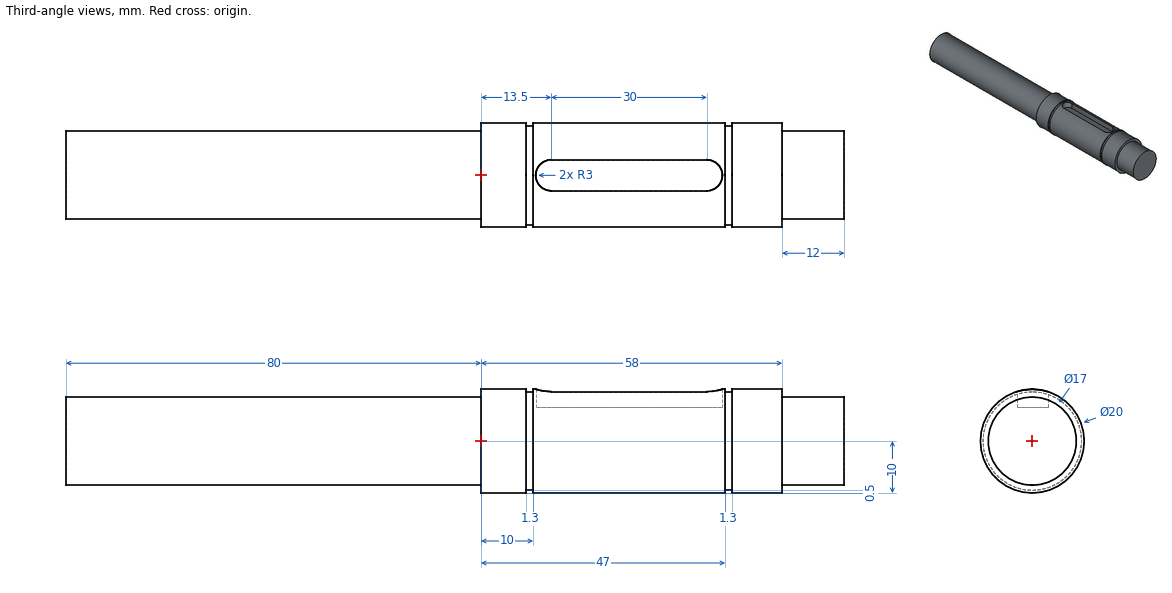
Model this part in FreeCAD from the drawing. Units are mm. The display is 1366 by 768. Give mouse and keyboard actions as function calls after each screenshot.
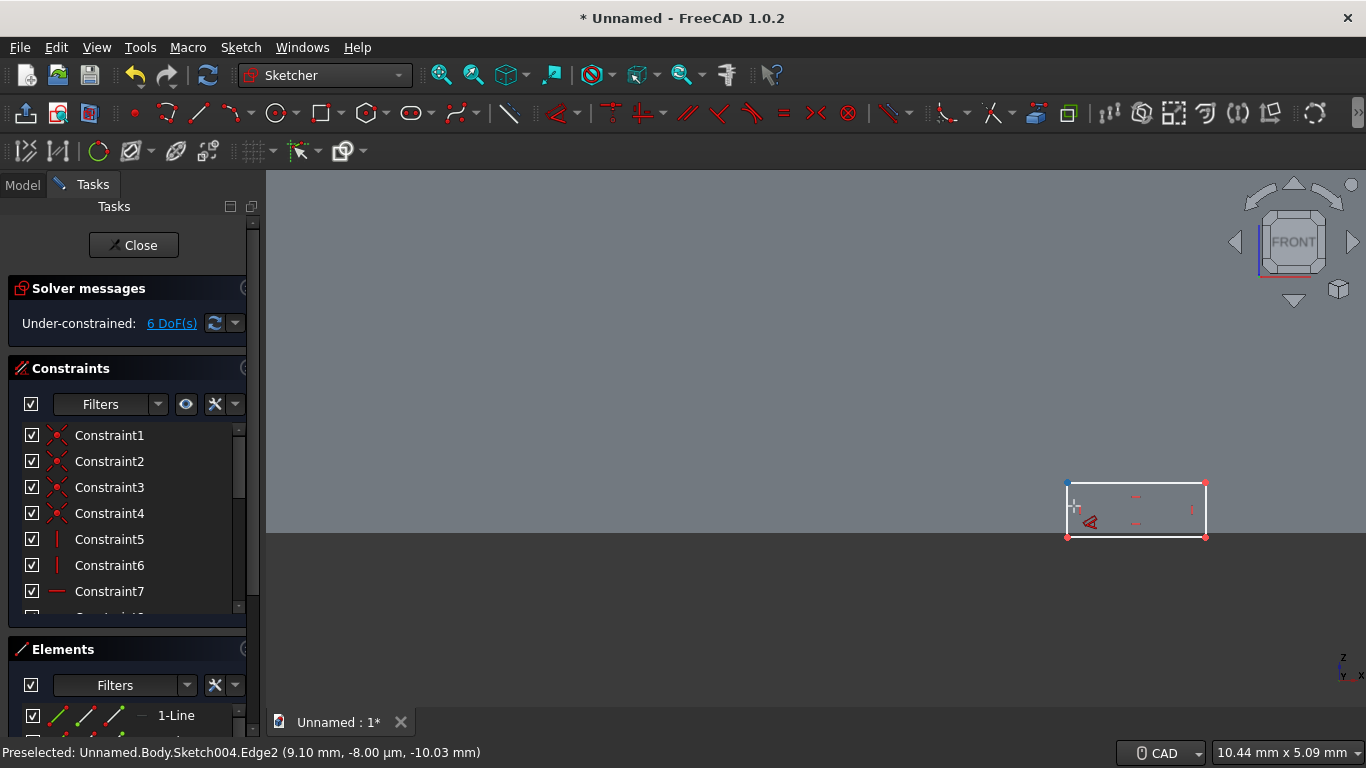
click(1067, 499)
click(1101, 510)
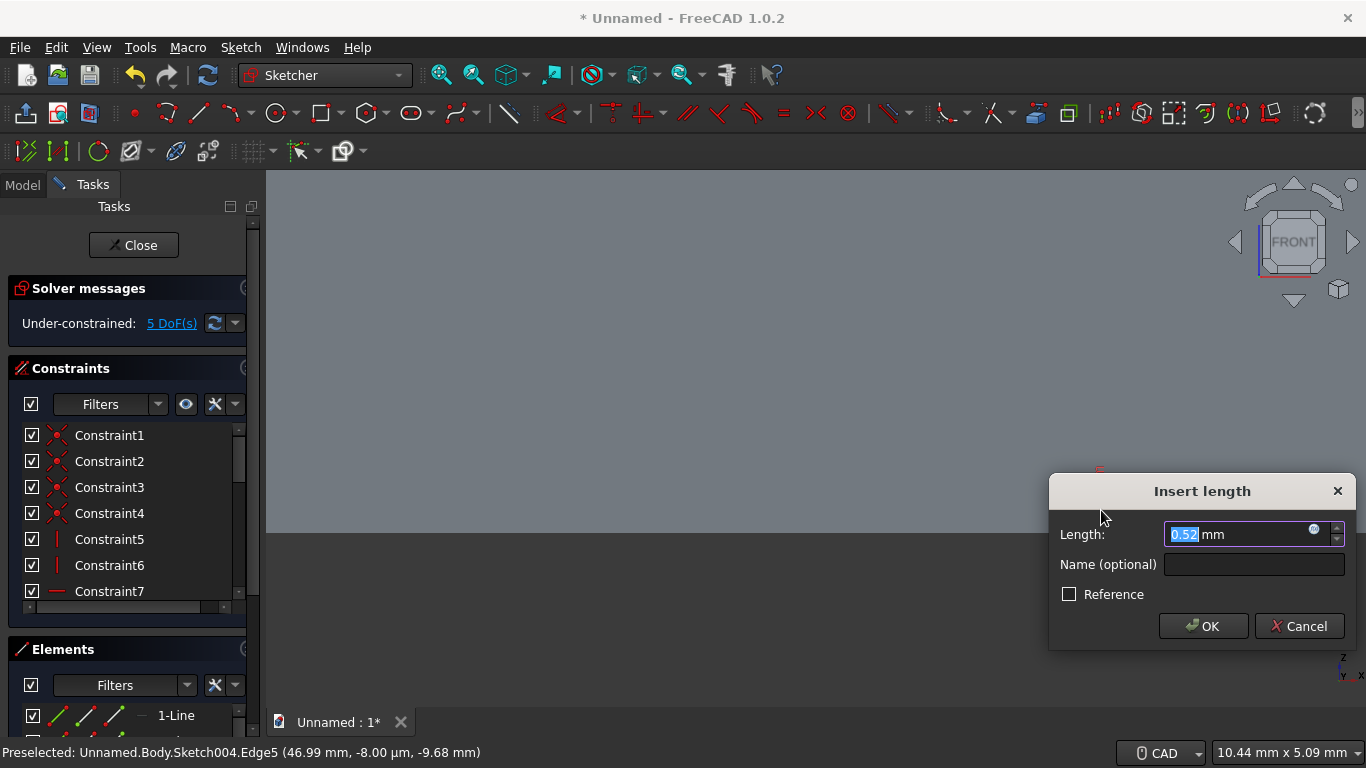
text(0.5)
key(Return)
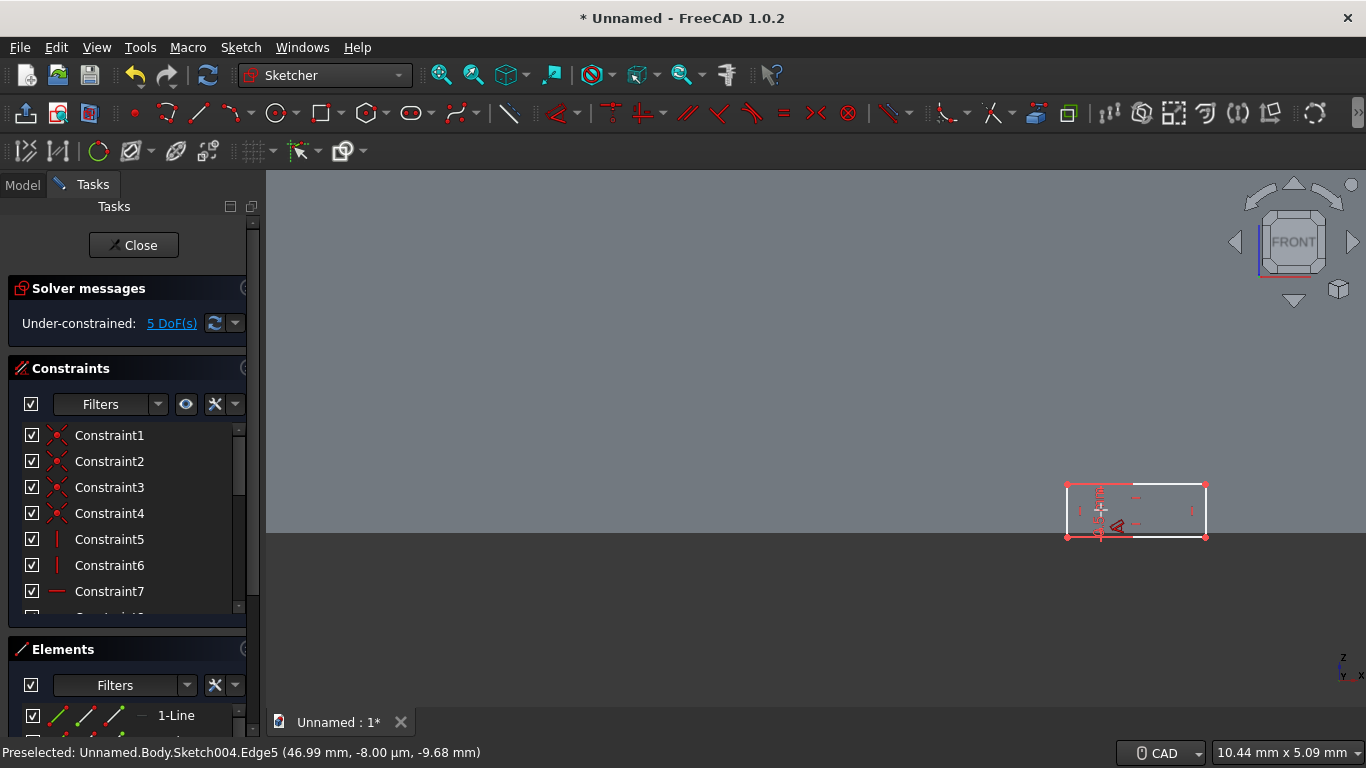
scroll(1074, 506, down, 10)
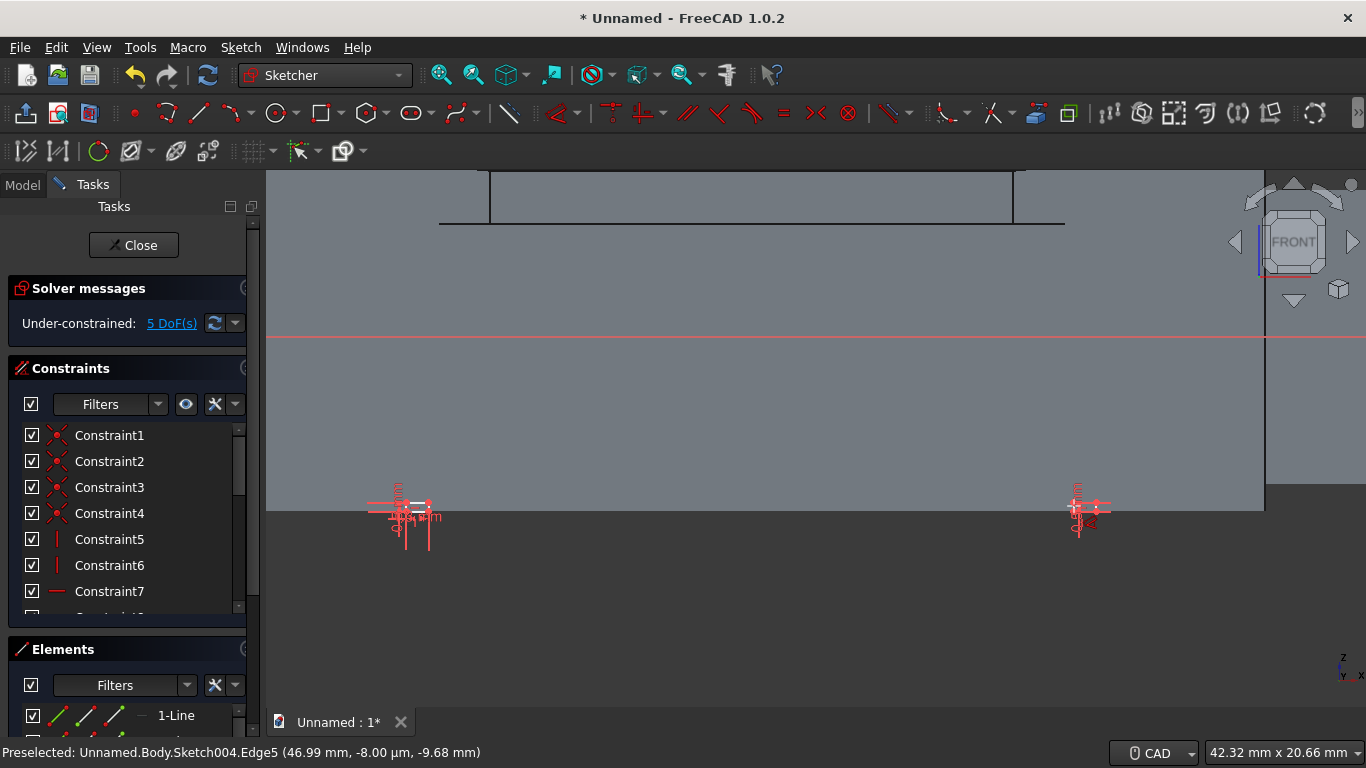
scroll(1079, 511, up, 5)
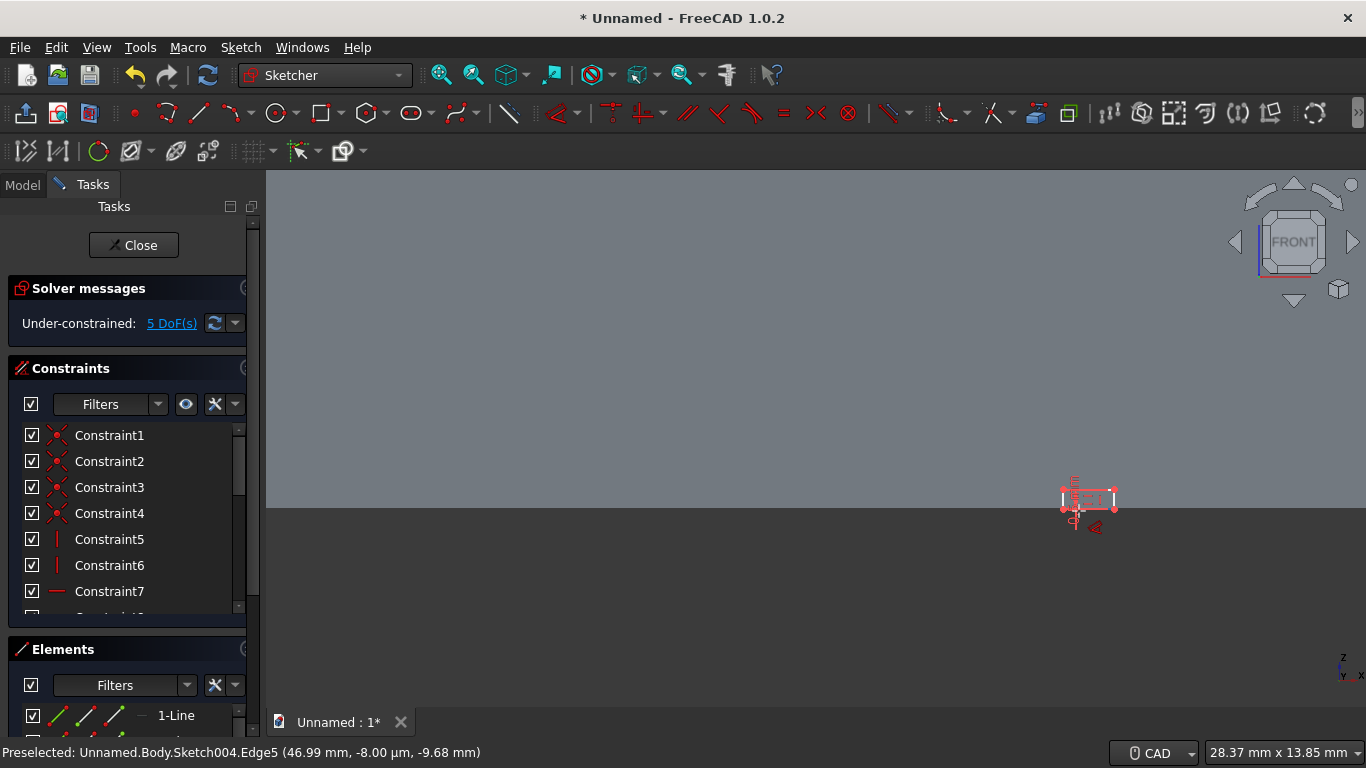
click(1079, 509)
click(1089, 543)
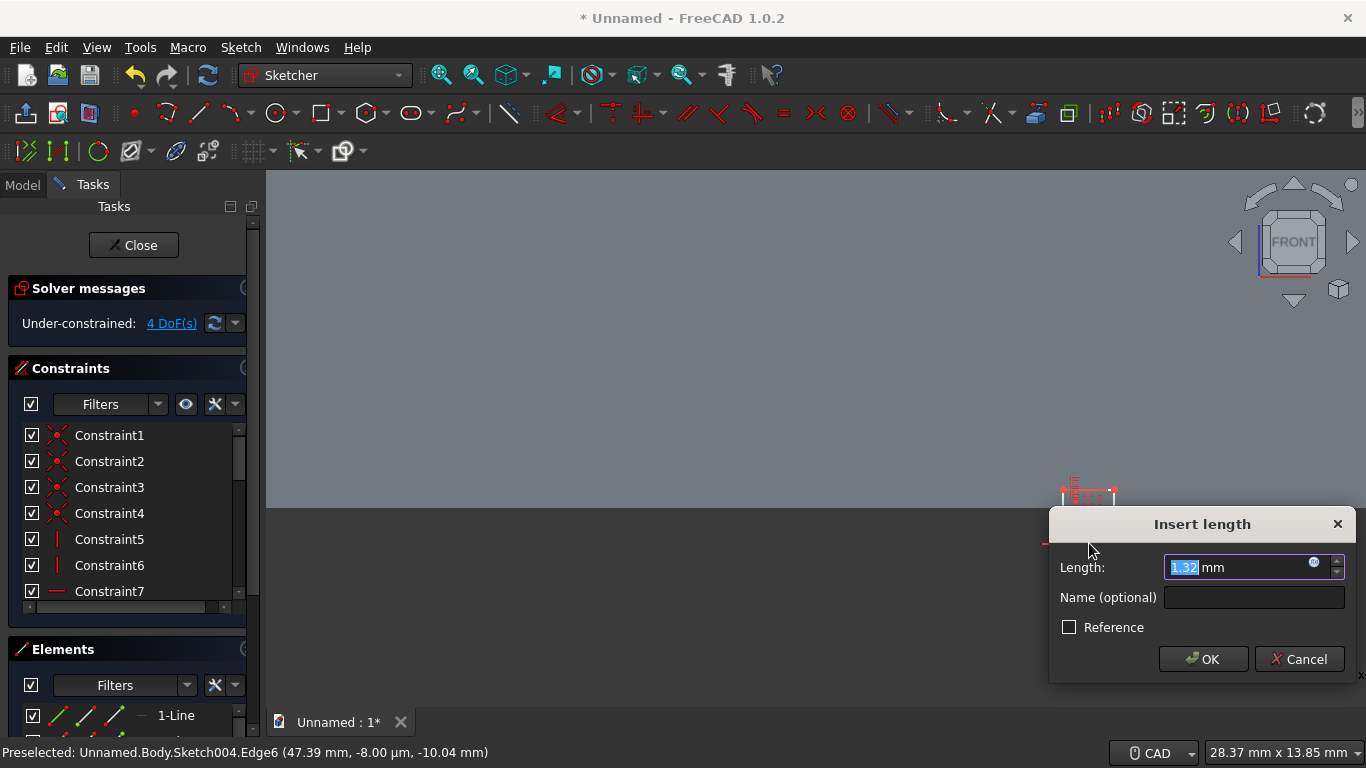
text(1.3)
key(Return)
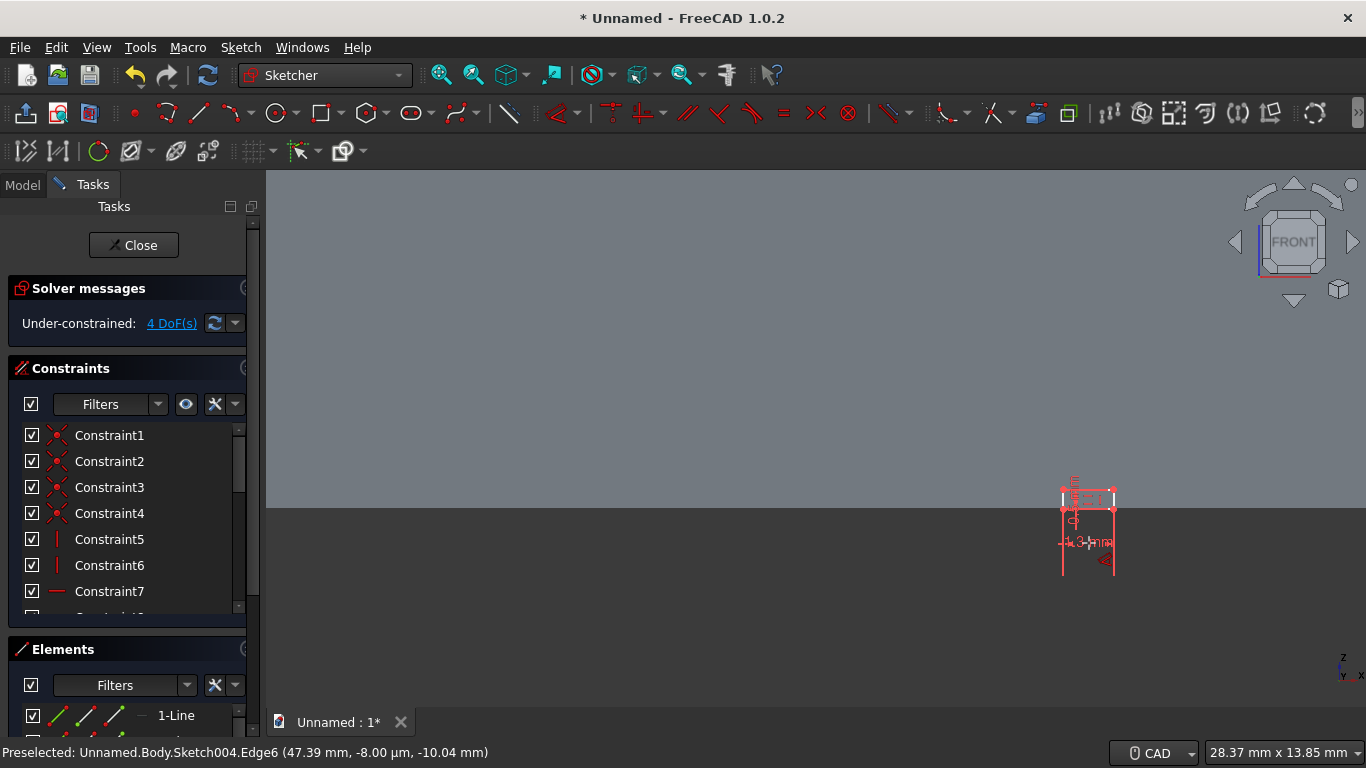
scroll(1079, 511, down, 5)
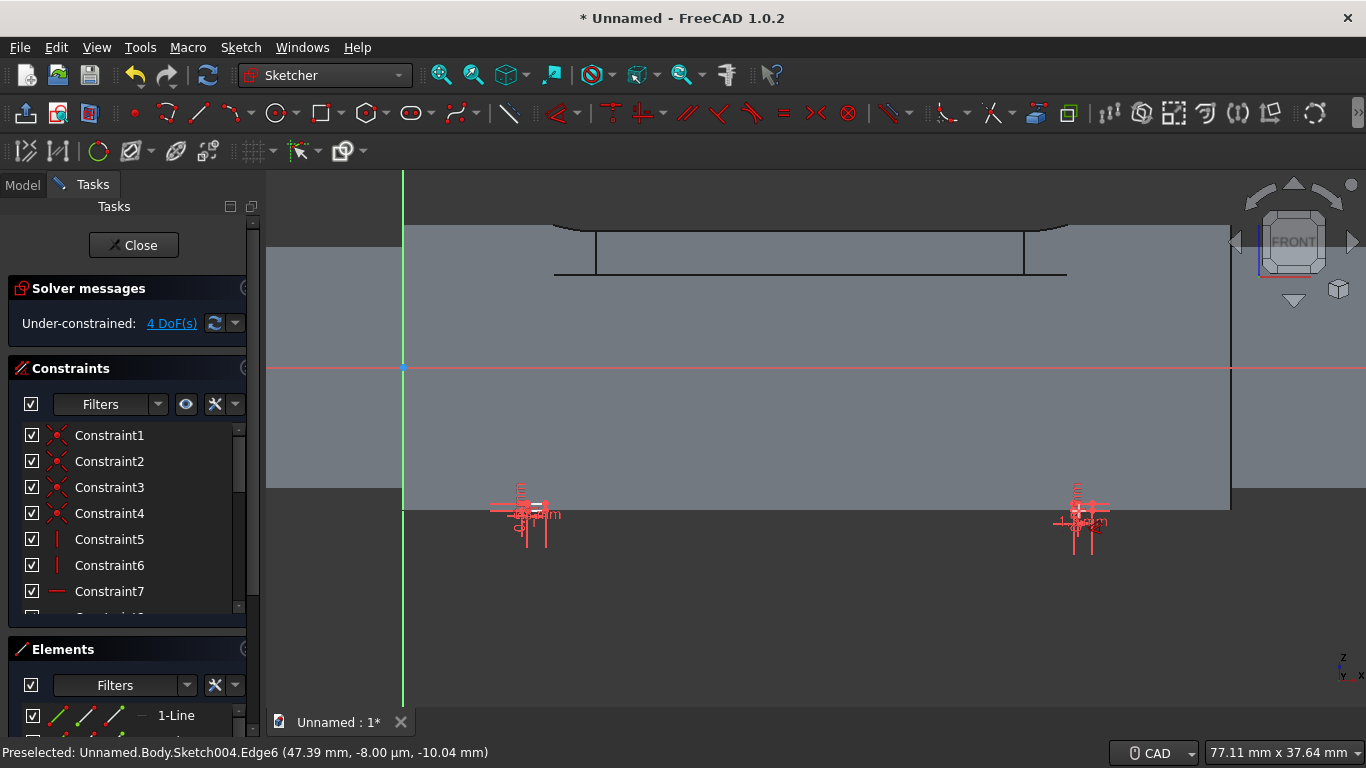
scroll(527, 511, up, 3)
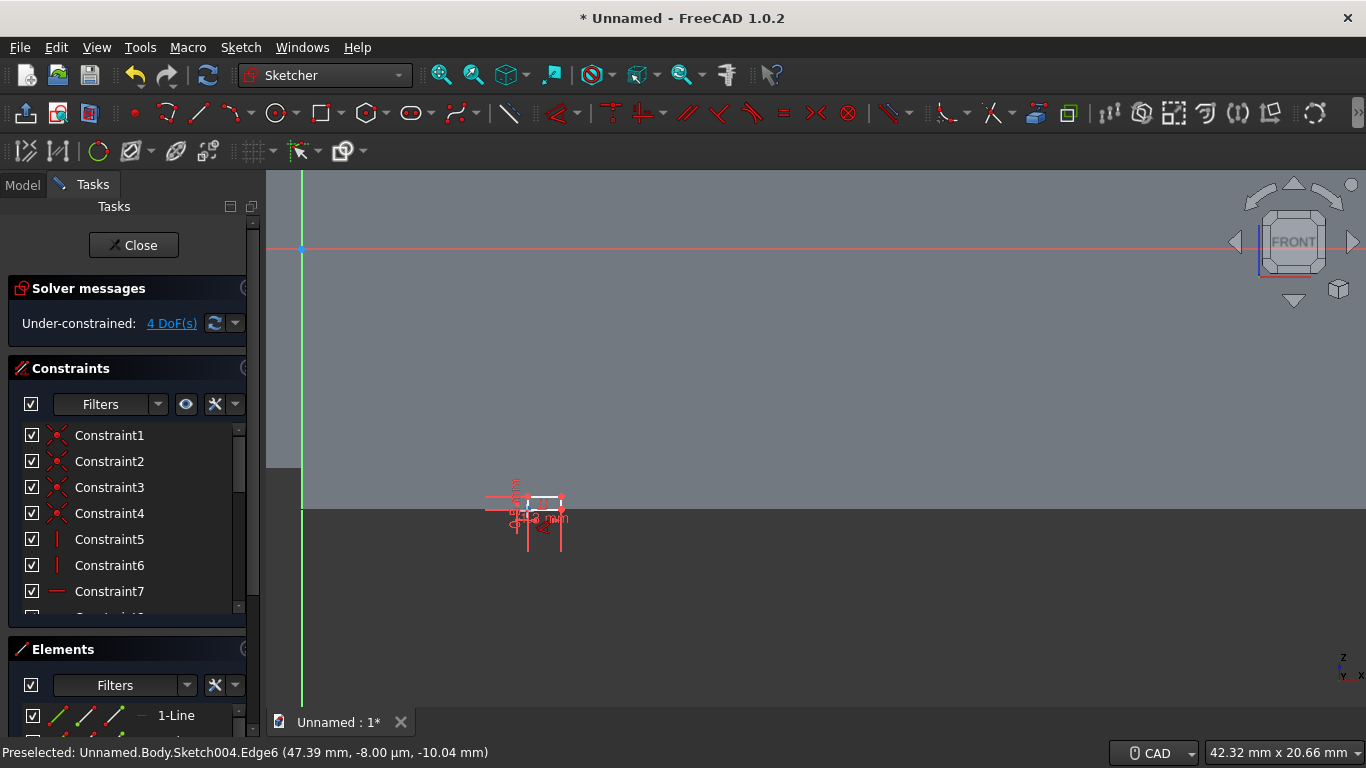
click(528, 510)
click(562, 380)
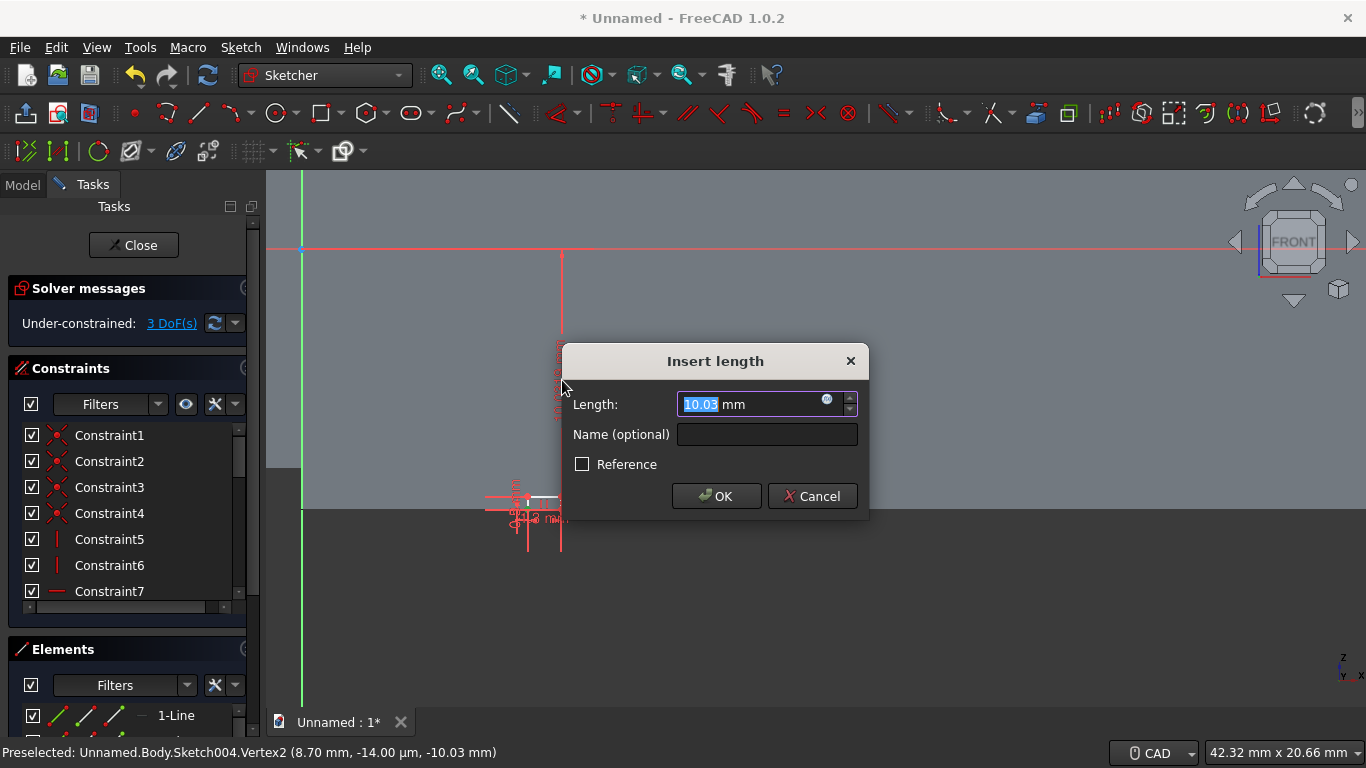
text(10)
key(Return)